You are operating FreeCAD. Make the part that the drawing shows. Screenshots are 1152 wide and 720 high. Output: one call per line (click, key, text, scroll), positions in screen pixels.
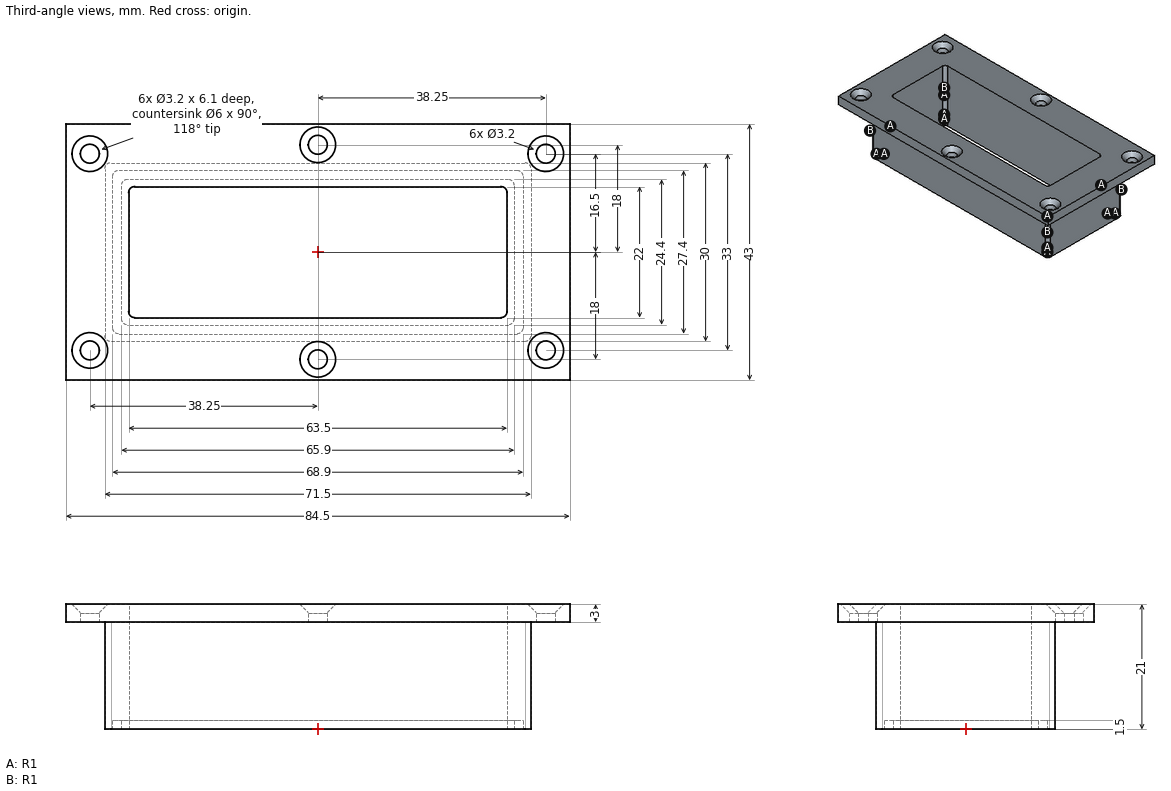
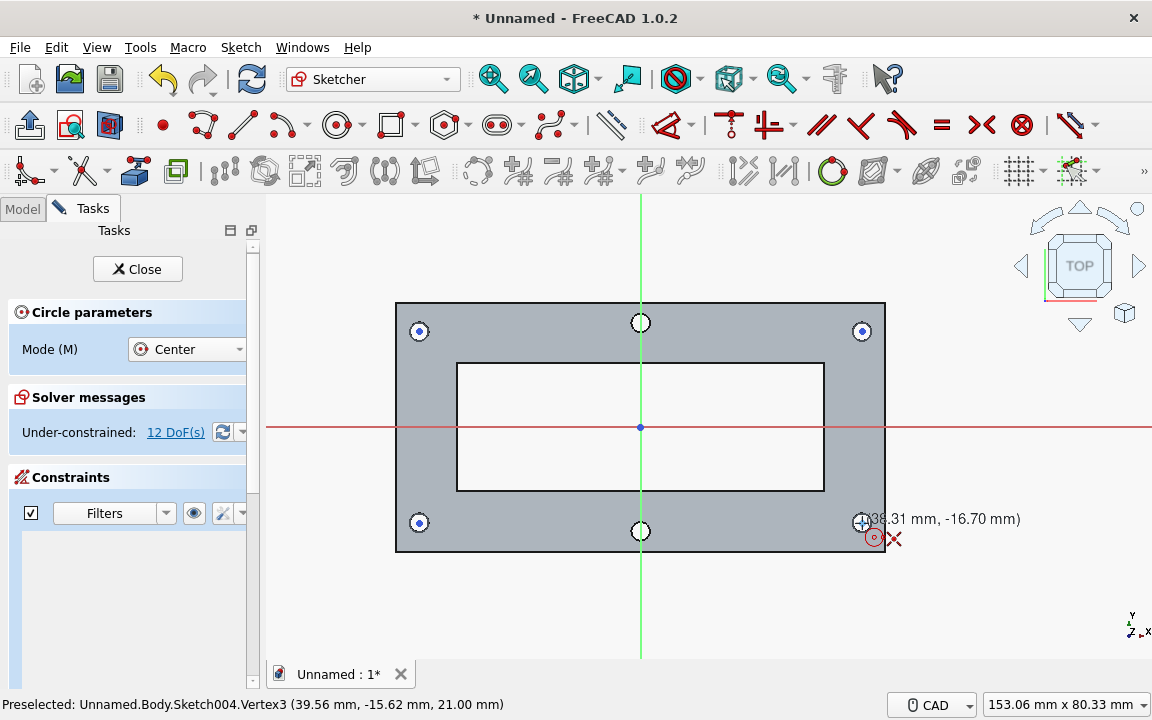
scroll(641, 531, up, 5)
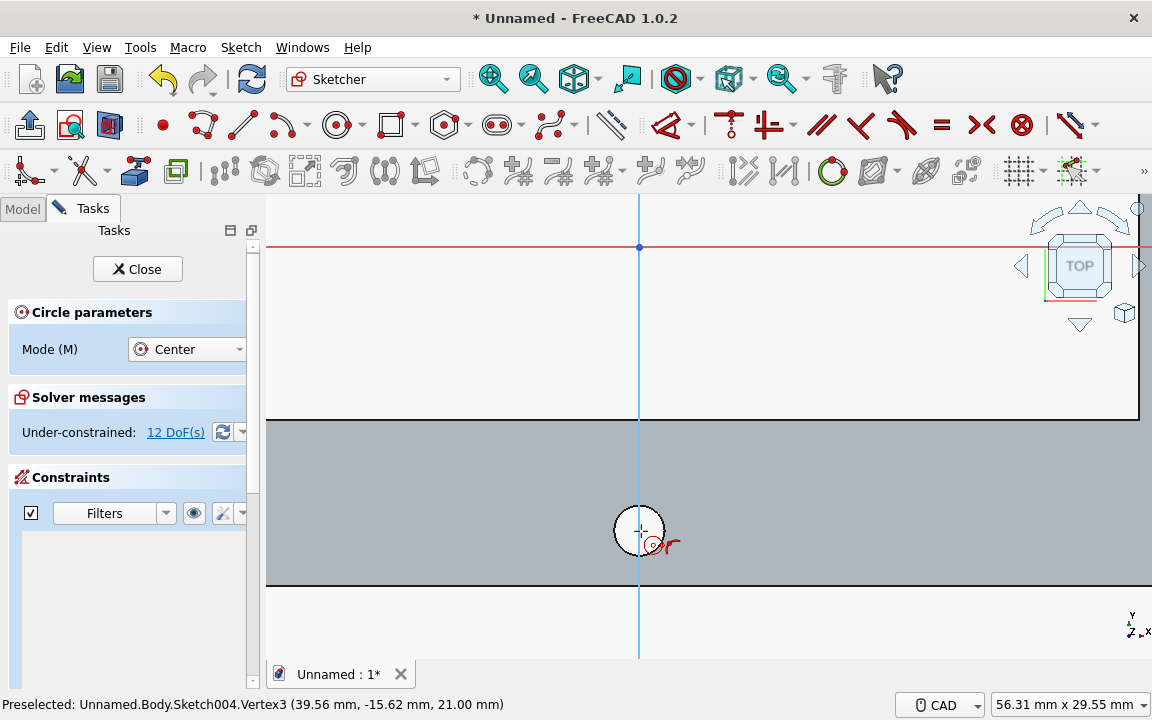
click(639, 531)
click(657, 513)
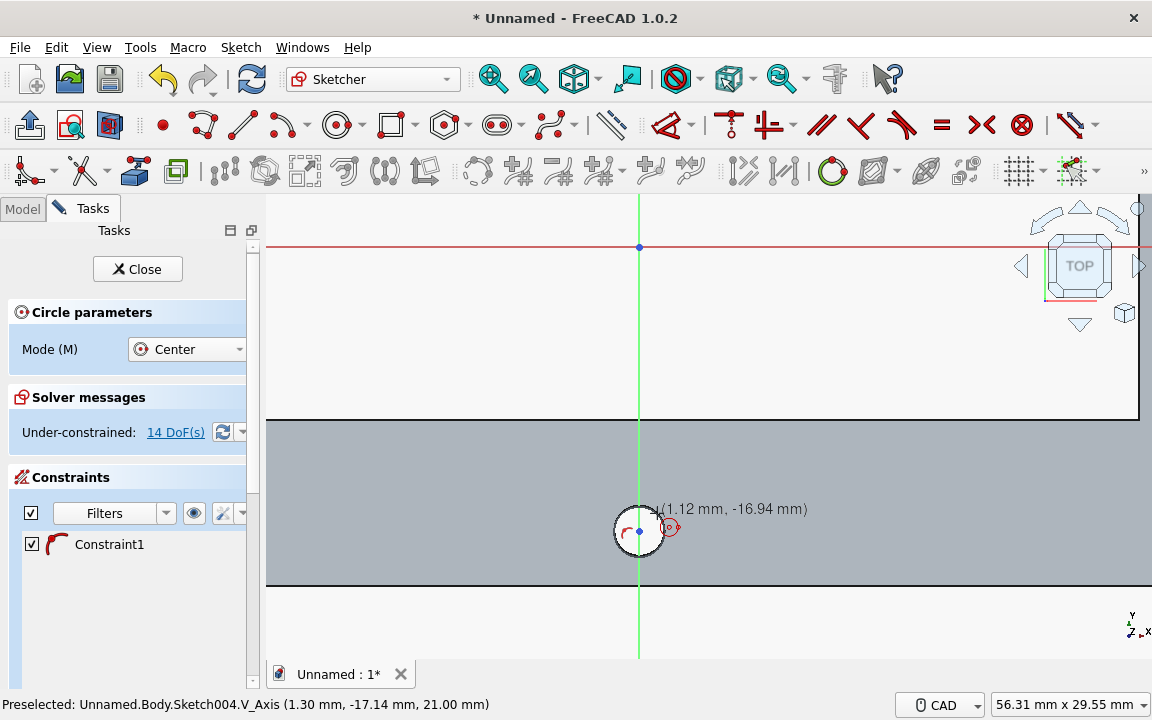
scroll(641, 531, down, 5)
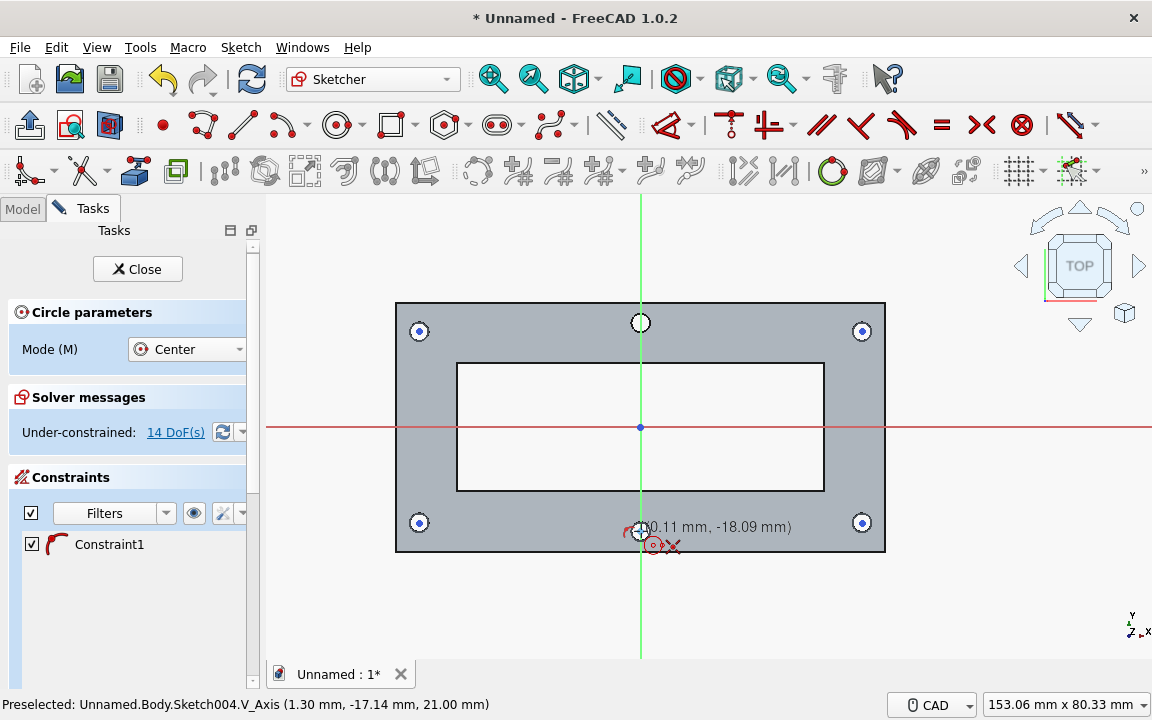
scroll(641, 323, up, 5)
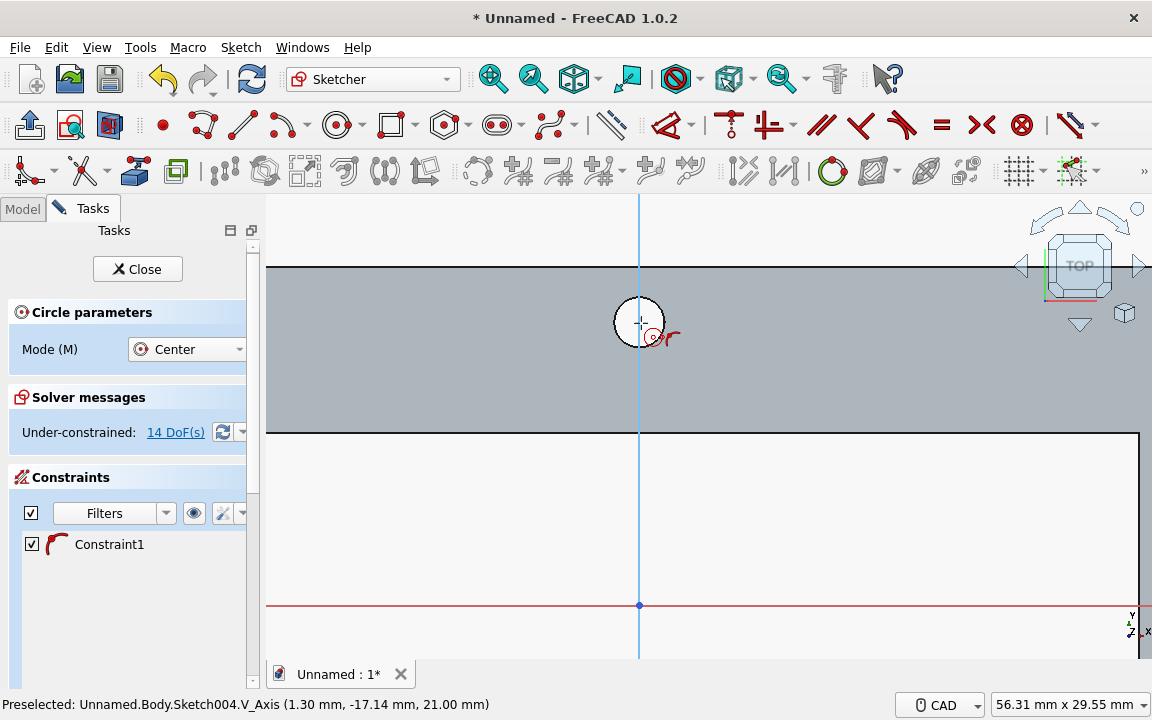
click(639, 322)
click(657, 305)
key(Escape)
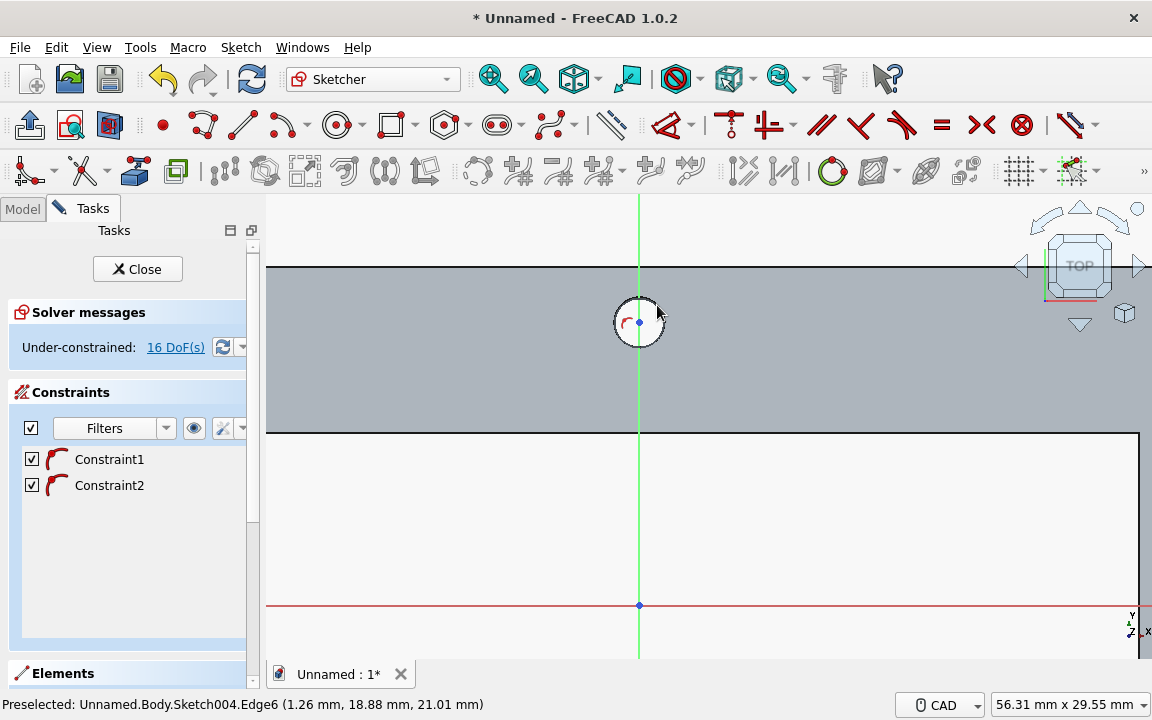
scroll(641, 322, down, 5)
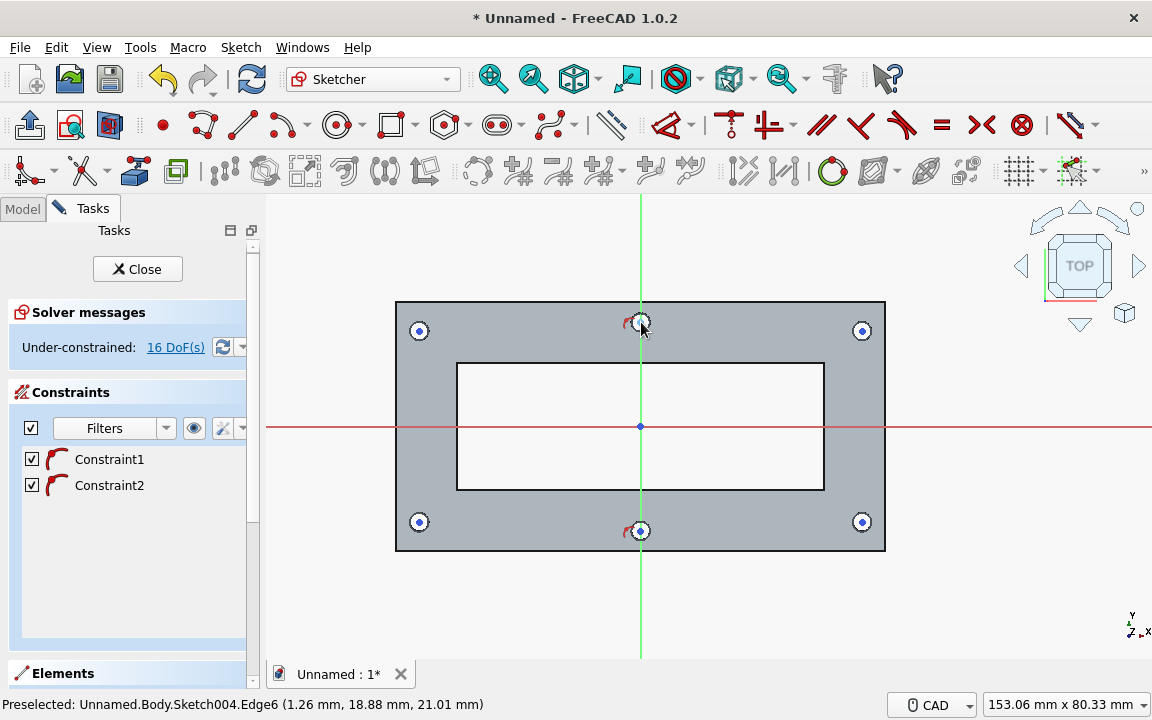
scroll(425, 325, up, 3)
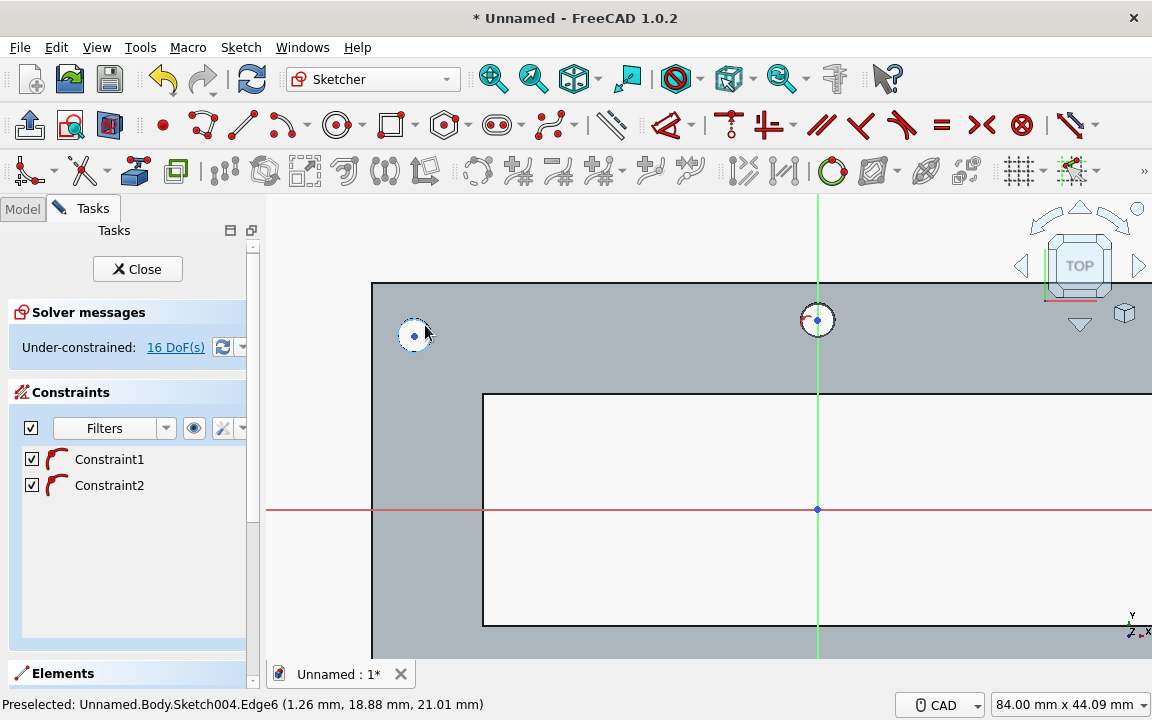
click(426, 324)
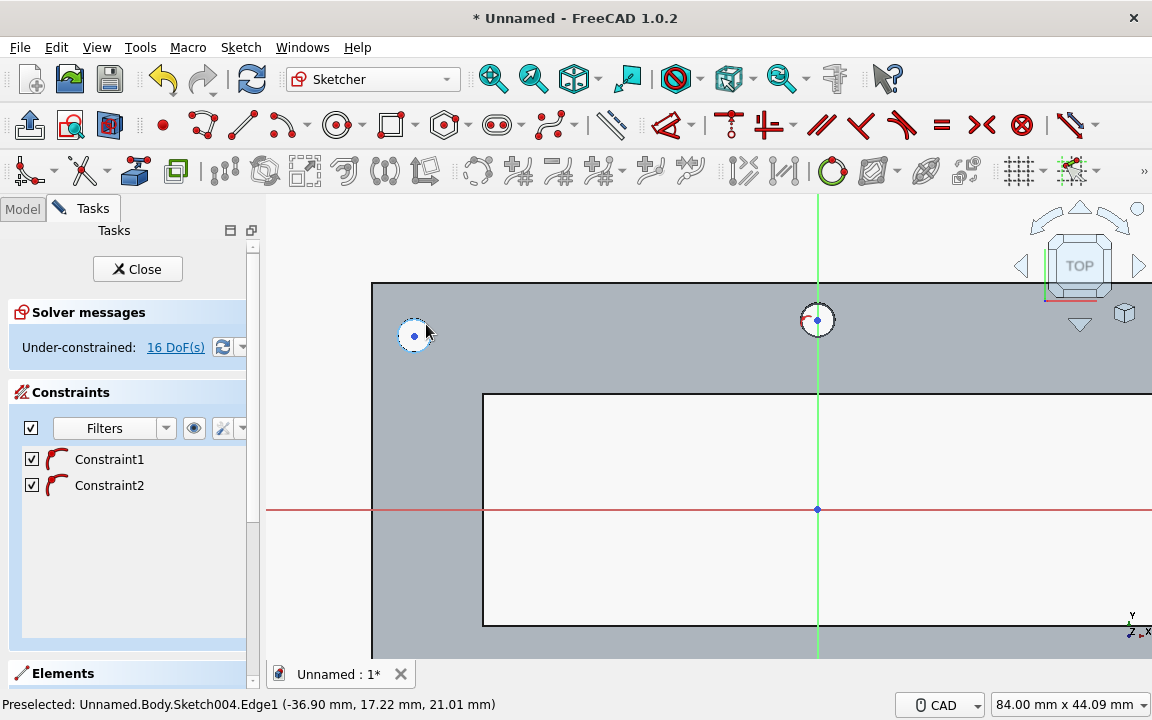
scroll(425, 325, down, 3)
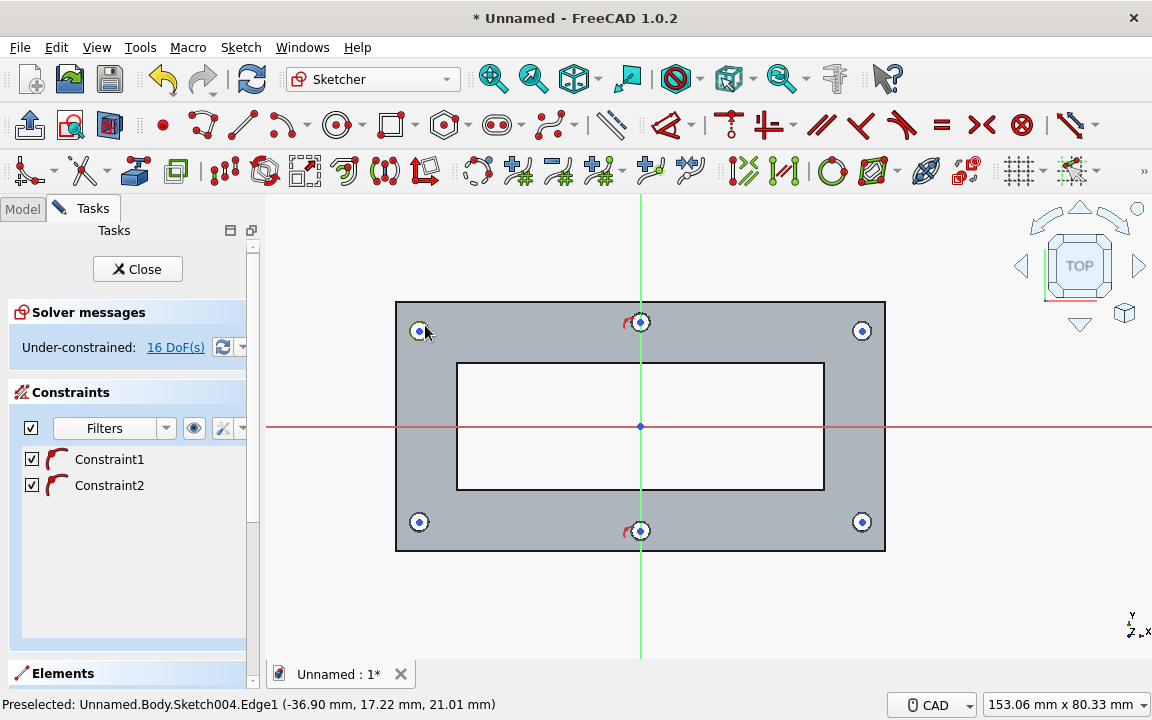
scroll(426, 516, up, 2)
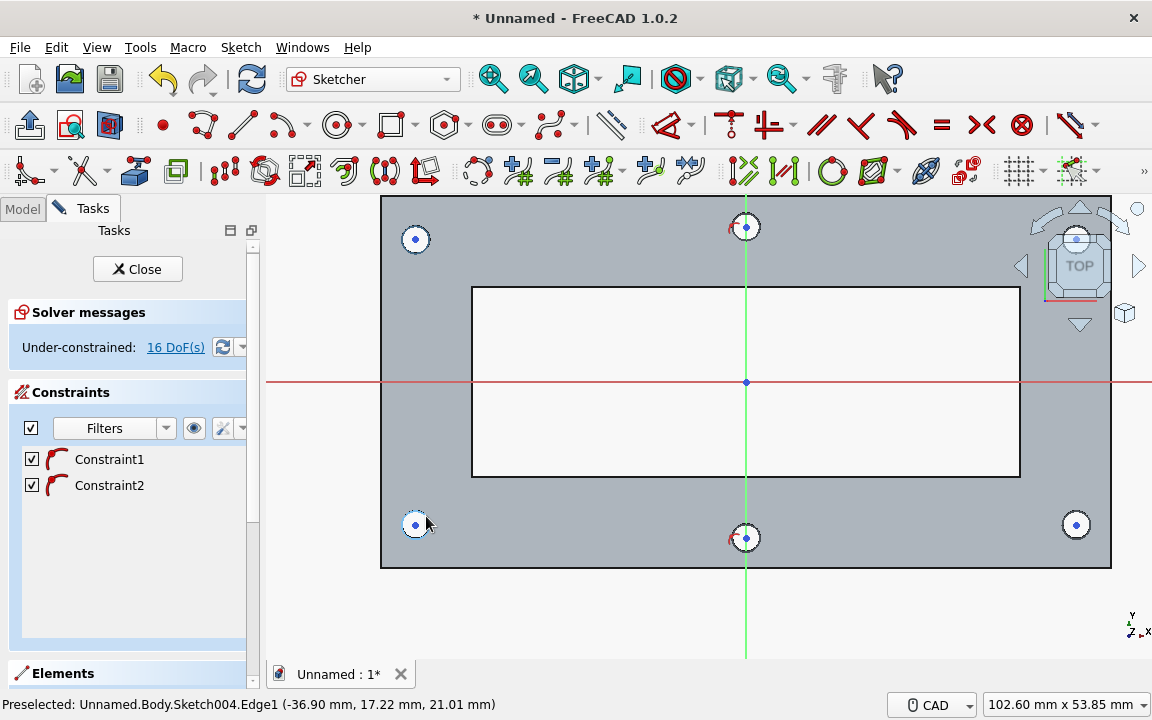
click(425, 515)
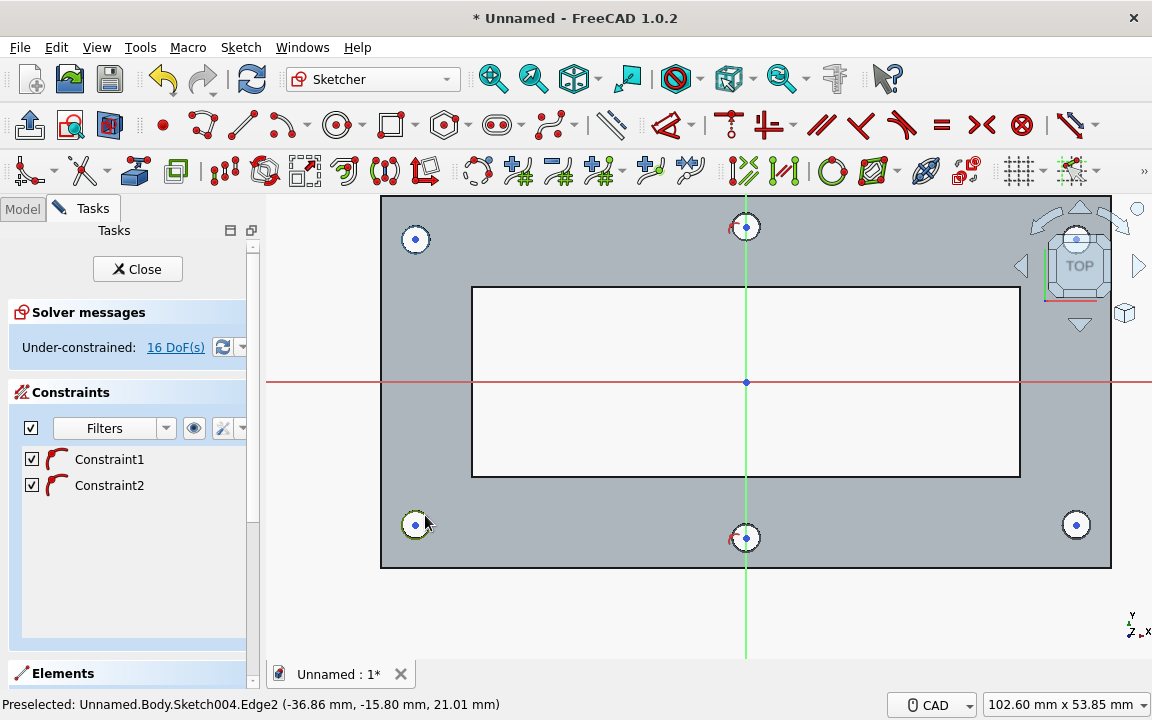
scroll(426, 517, down, 2)